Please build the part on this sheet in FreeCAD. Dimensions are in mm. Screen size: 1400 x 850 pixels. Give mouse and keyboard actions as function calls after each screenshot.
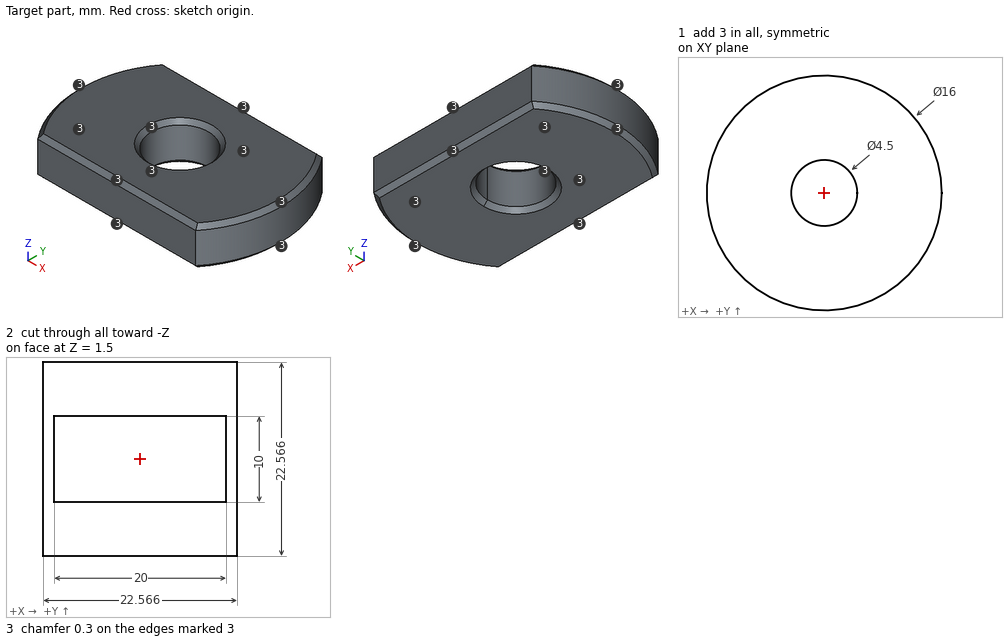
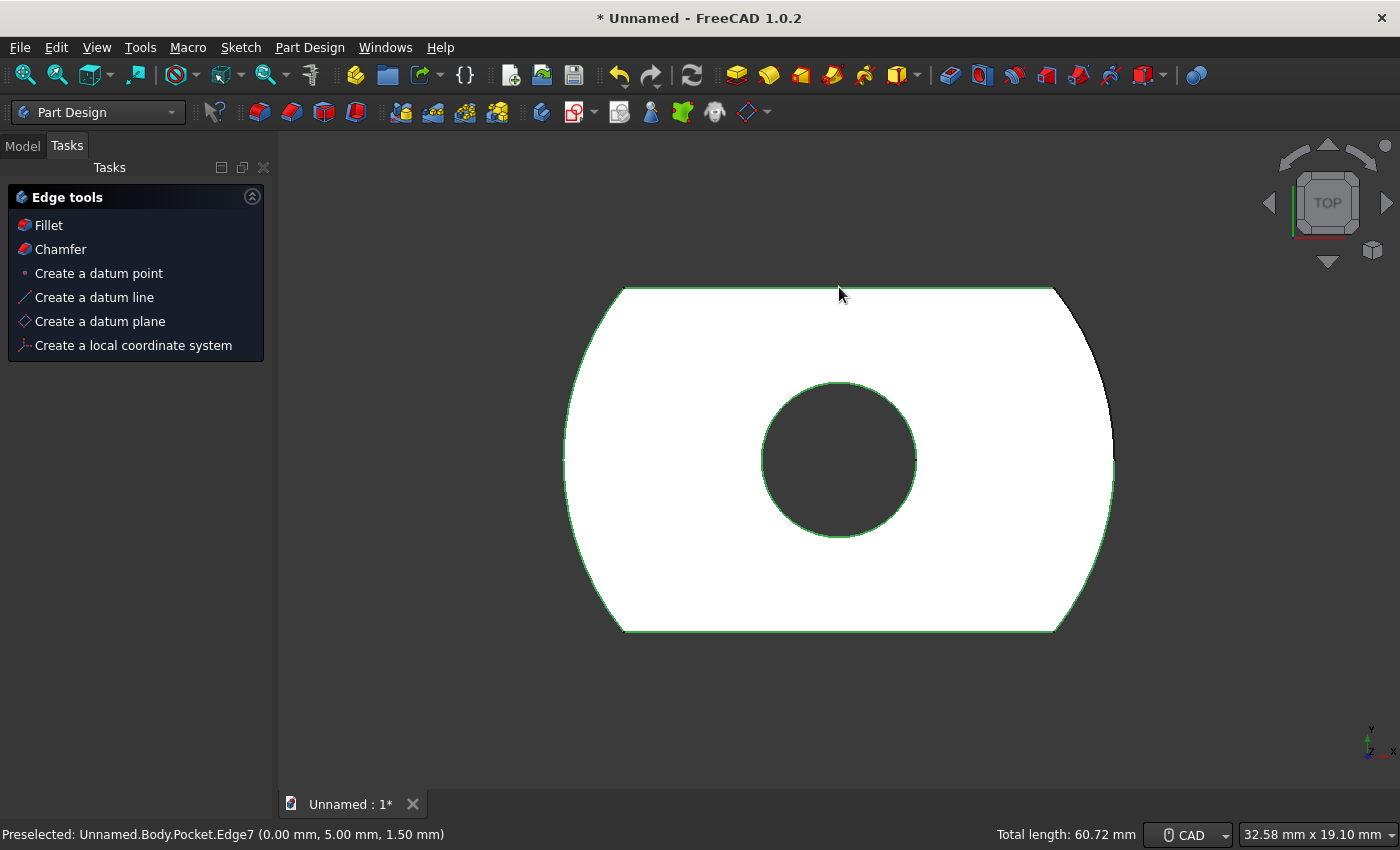
key(1)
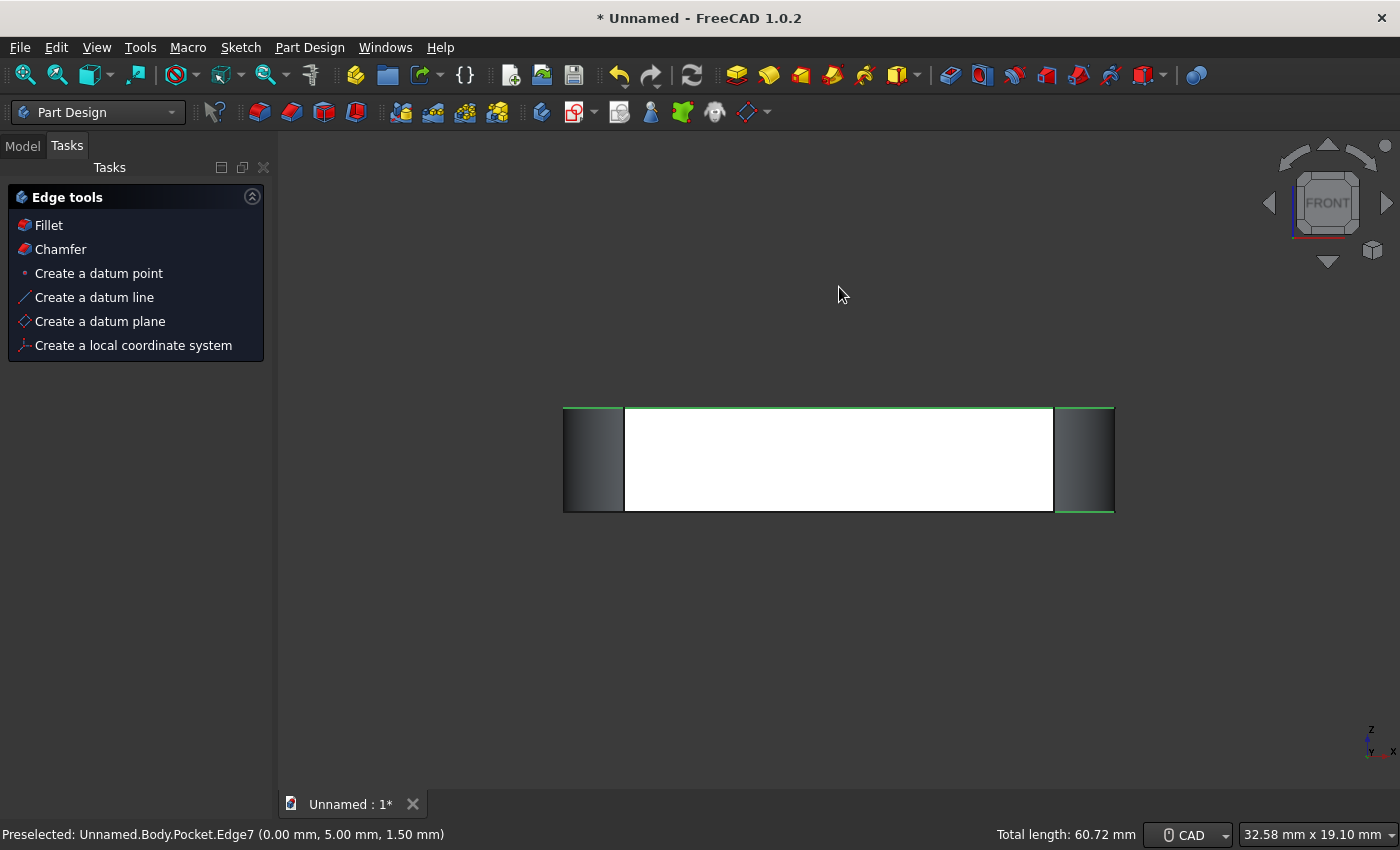
click(566, 511, ctrl)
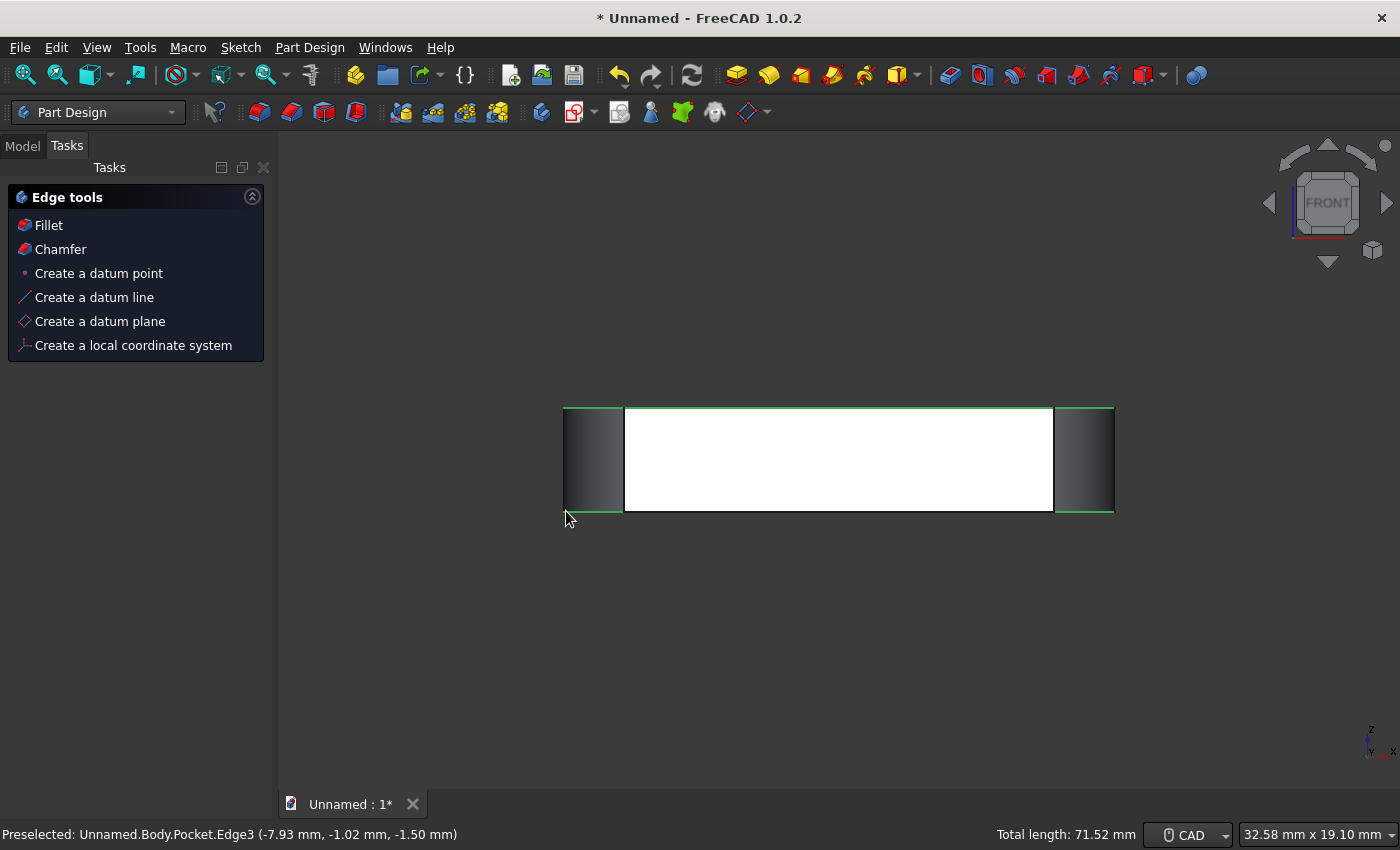
click(839, 511, ctrl)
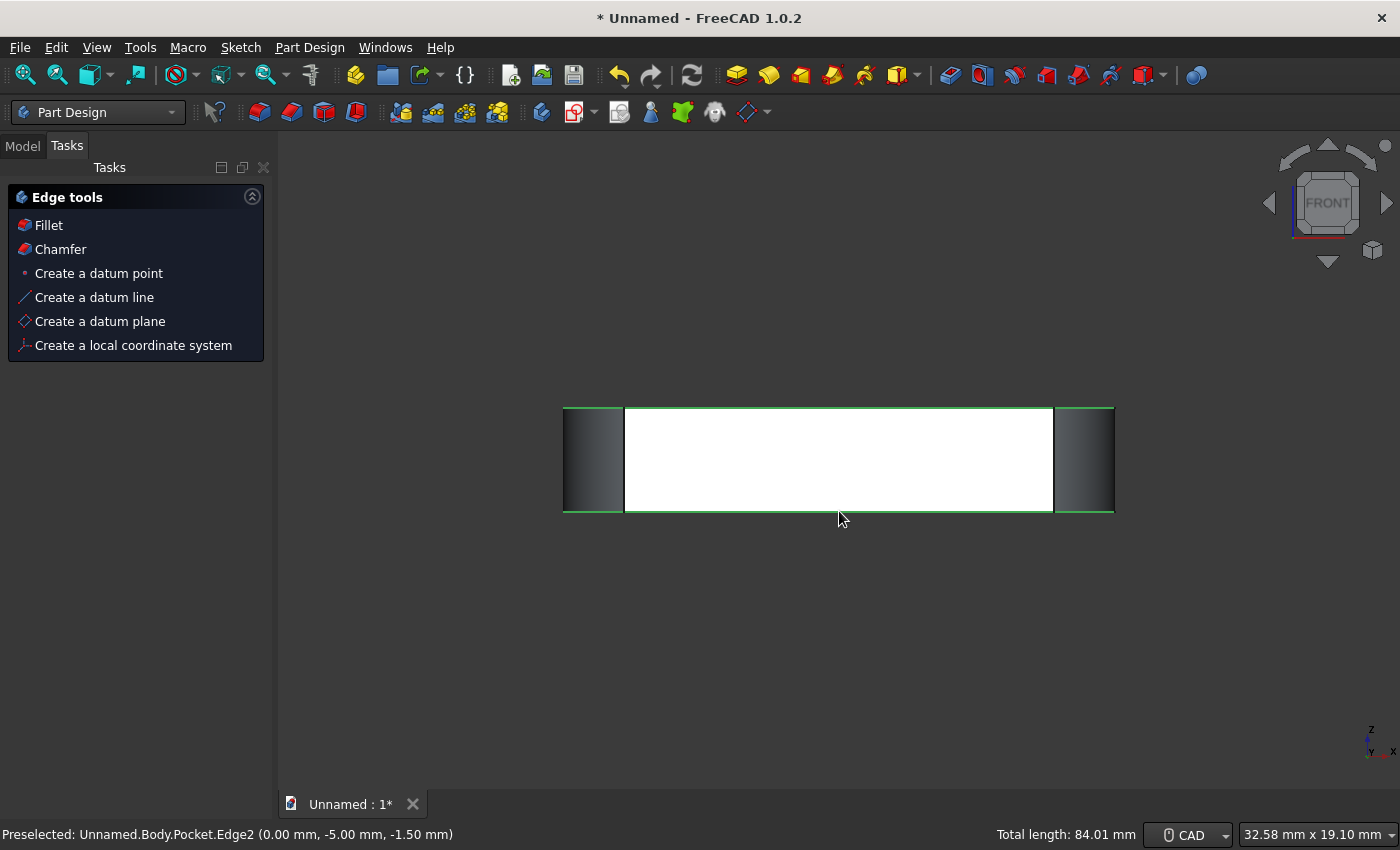
key(3)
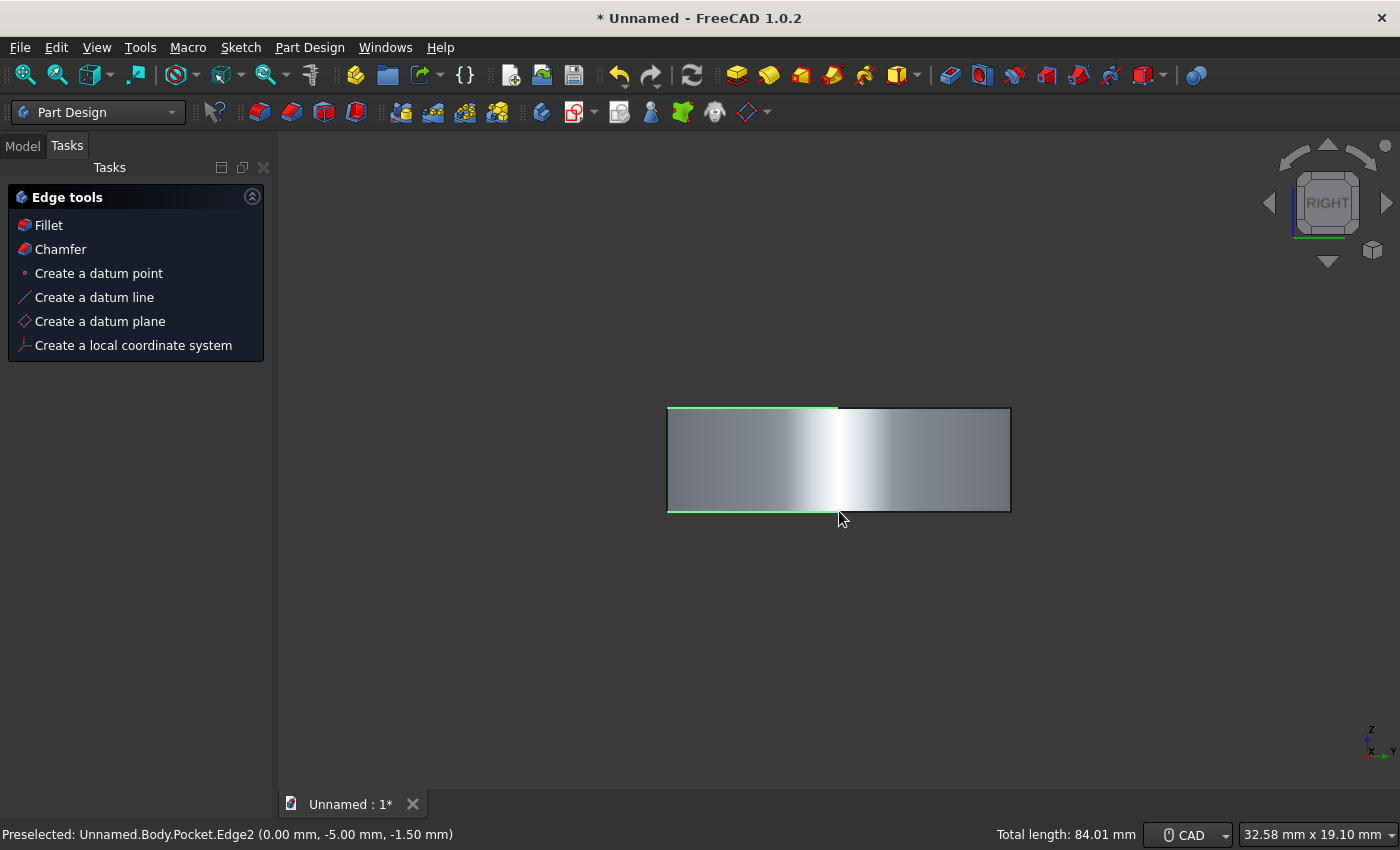
click(26, 76)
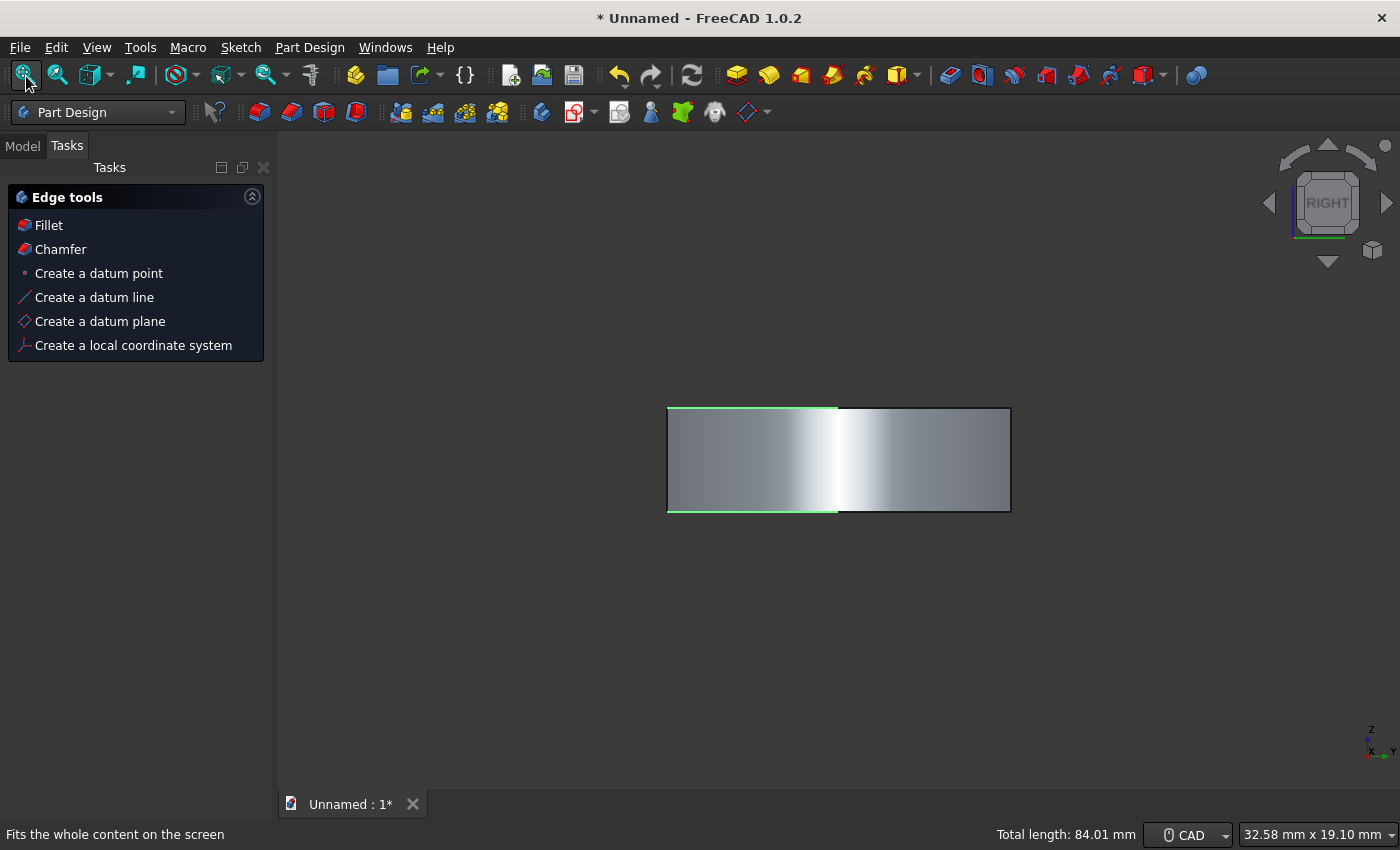
key(5)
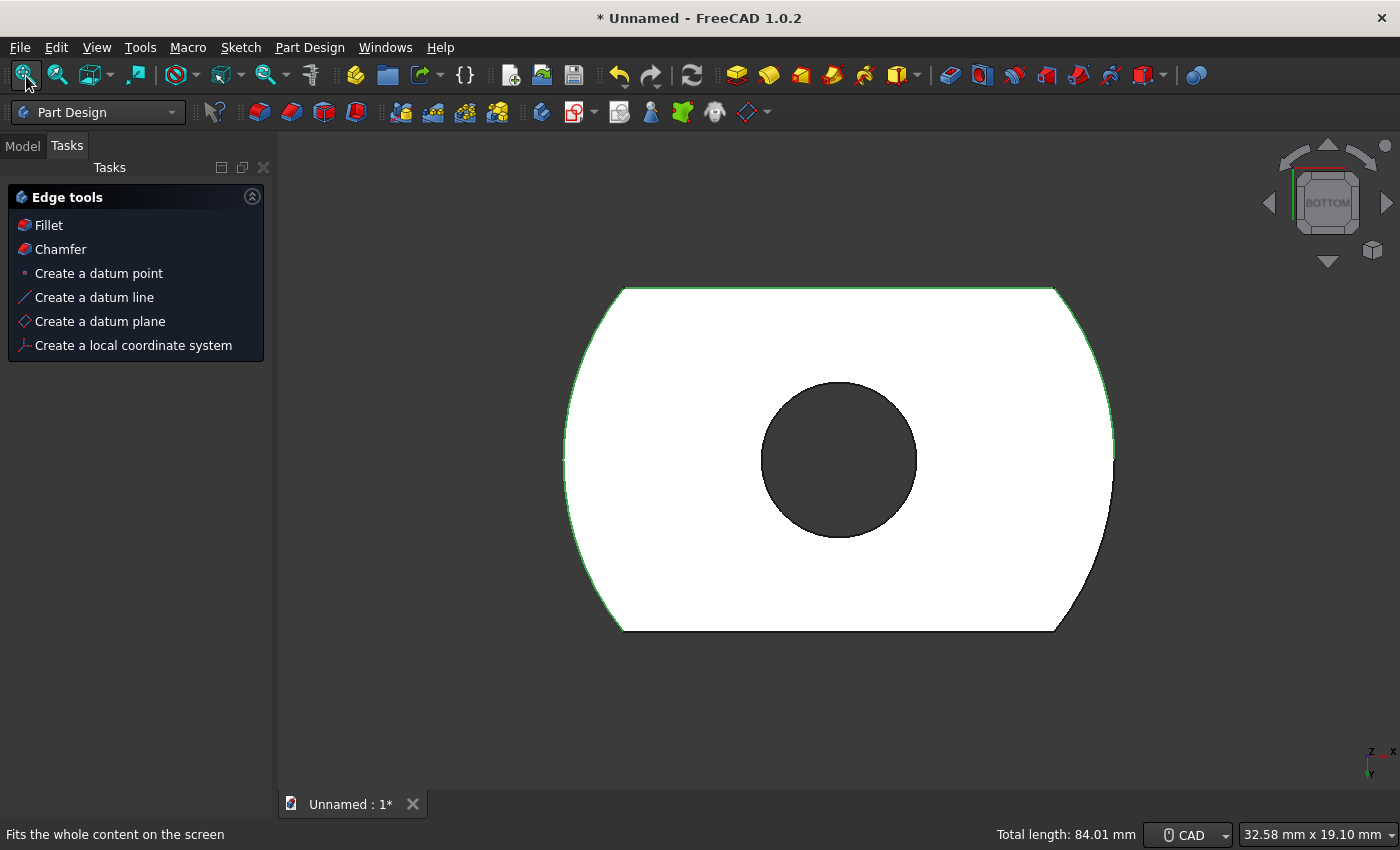
click(839, 631, ctrl)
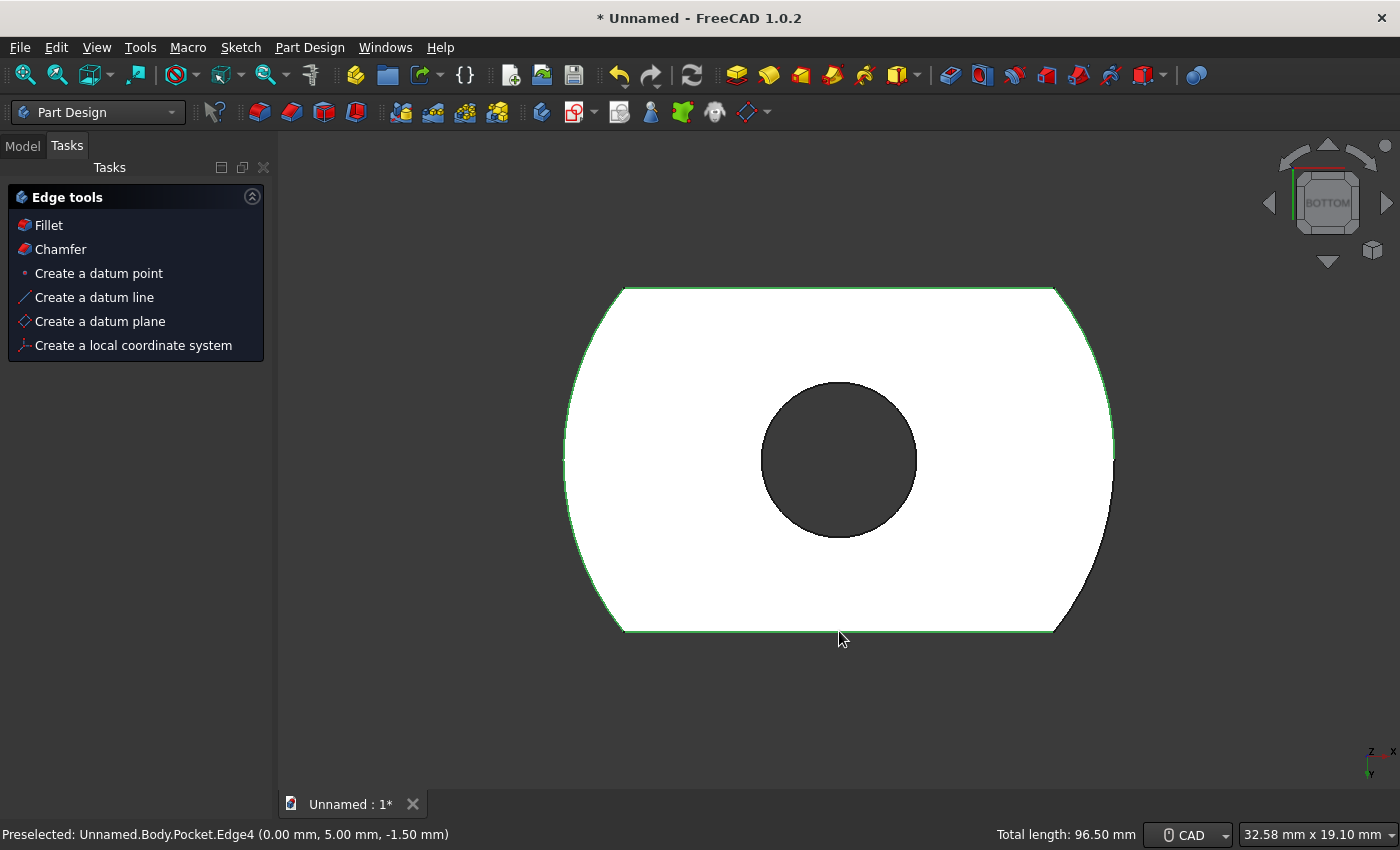
click(762, 459, ctrl)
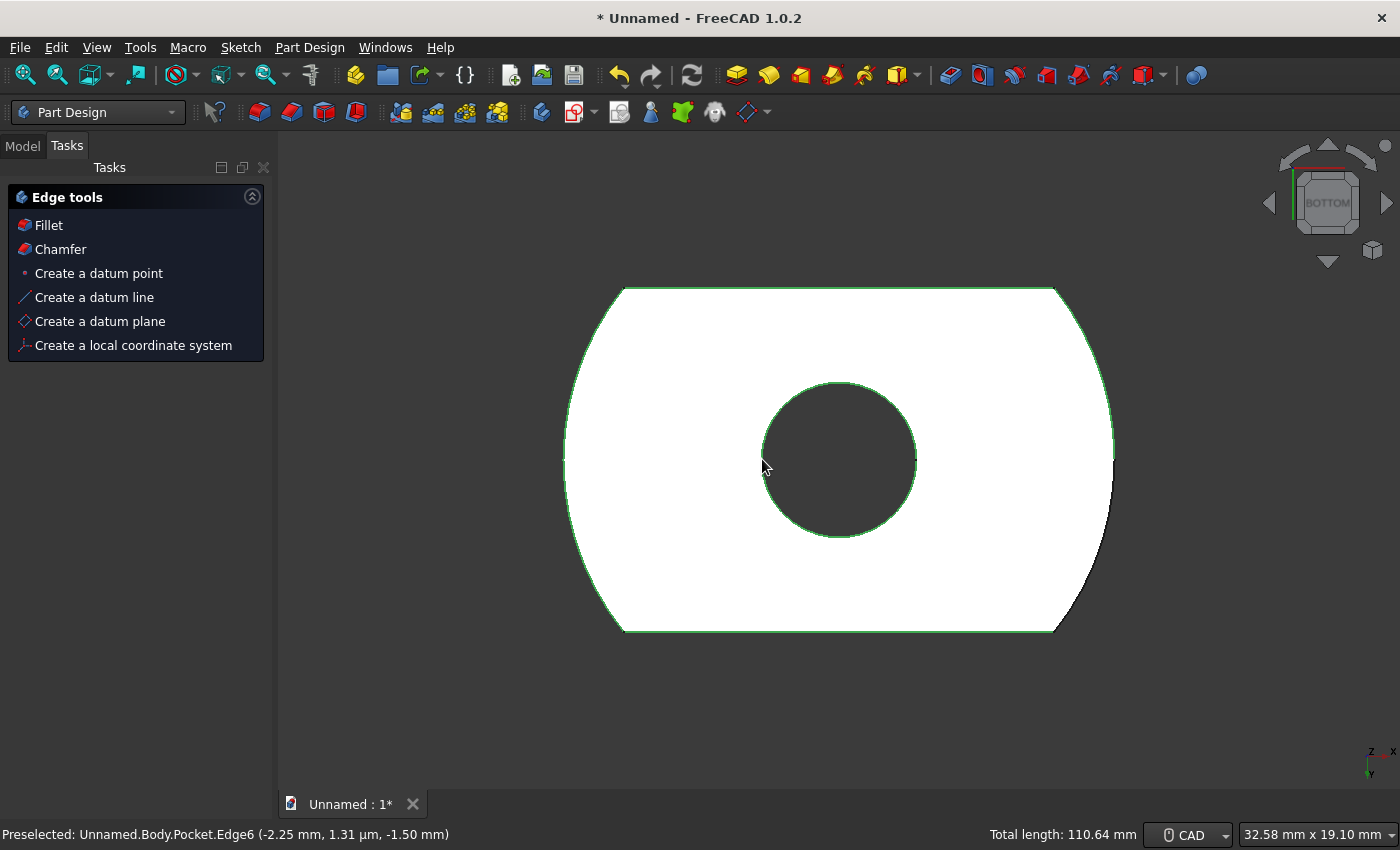
click(292, 112)